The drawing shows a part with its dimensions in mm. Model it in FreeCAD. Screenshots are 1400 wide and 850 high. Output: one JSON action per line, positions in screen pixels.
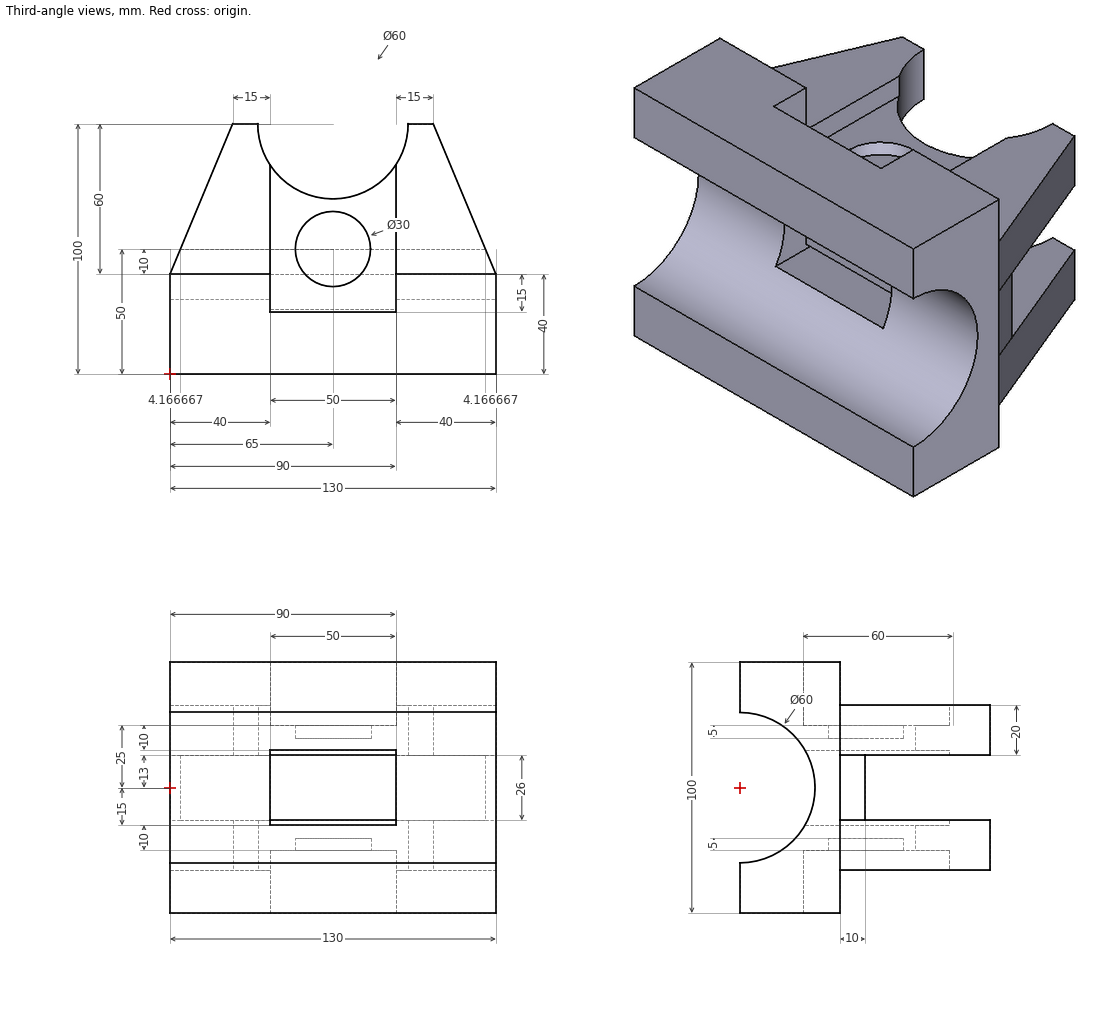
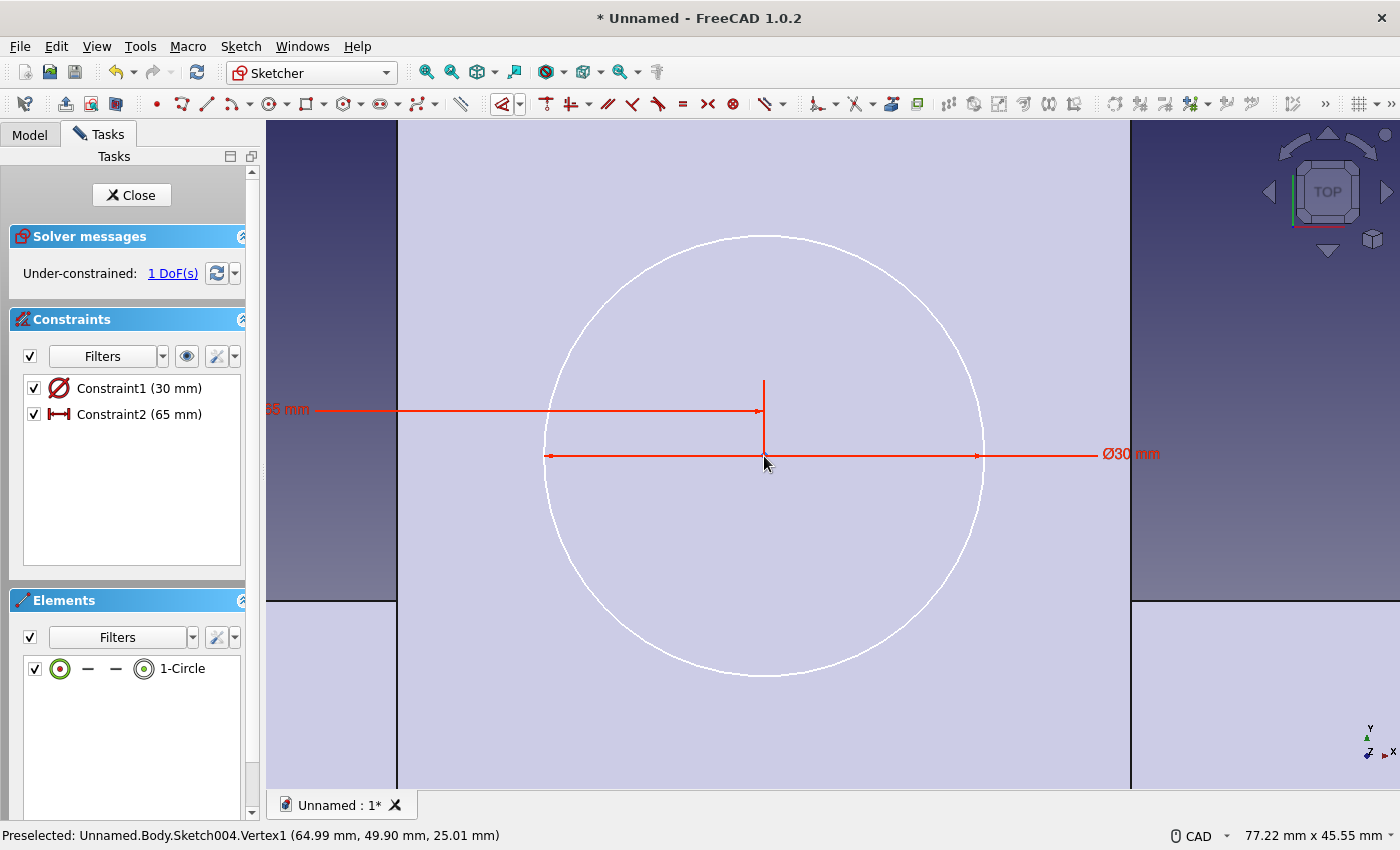
{"action": "left_click", "coordinate": [764, 456]}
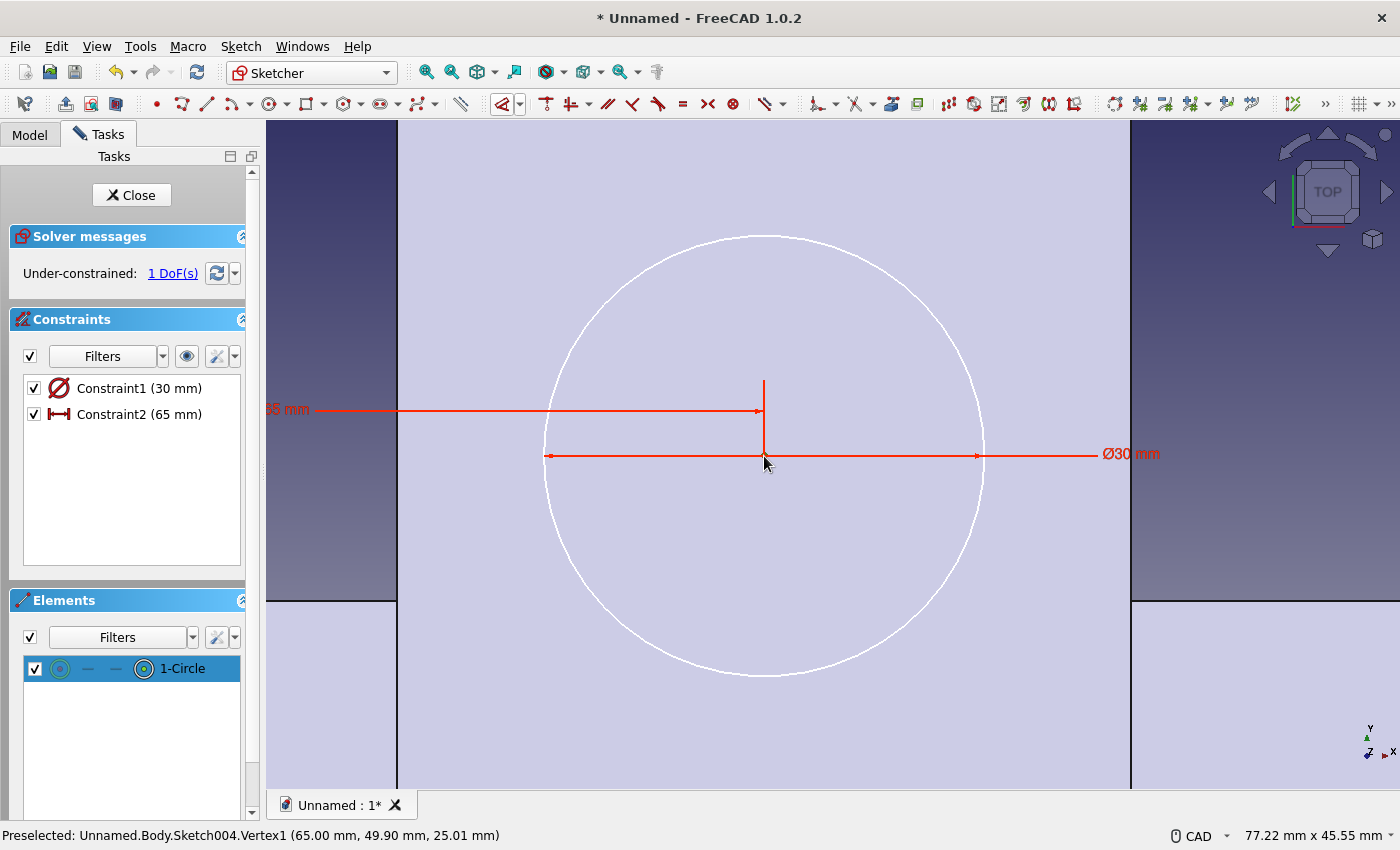
{"action": "key", "text": "i"}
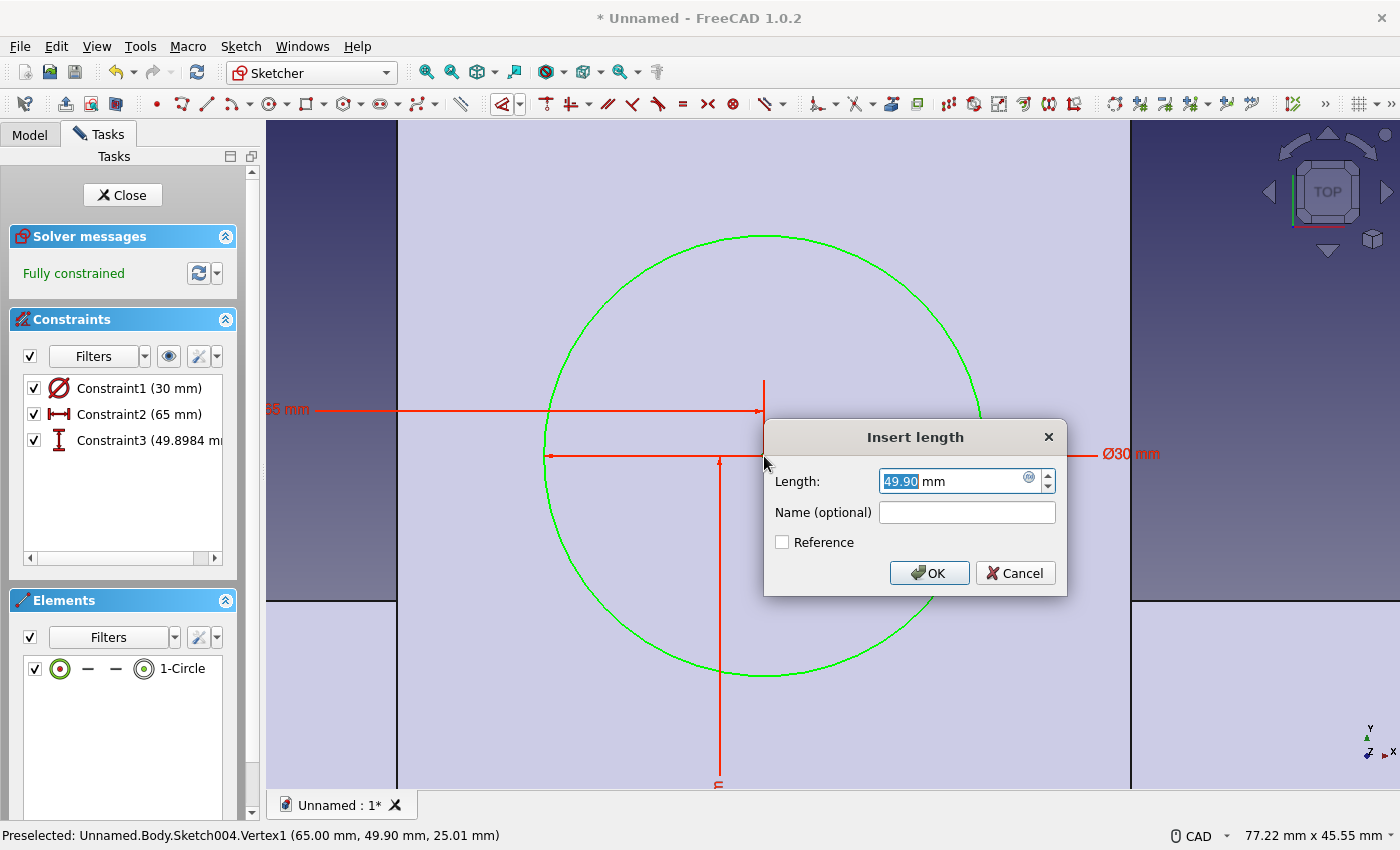
{"action": "type", "text": "50"}
{"action": "key", "text": "Return"}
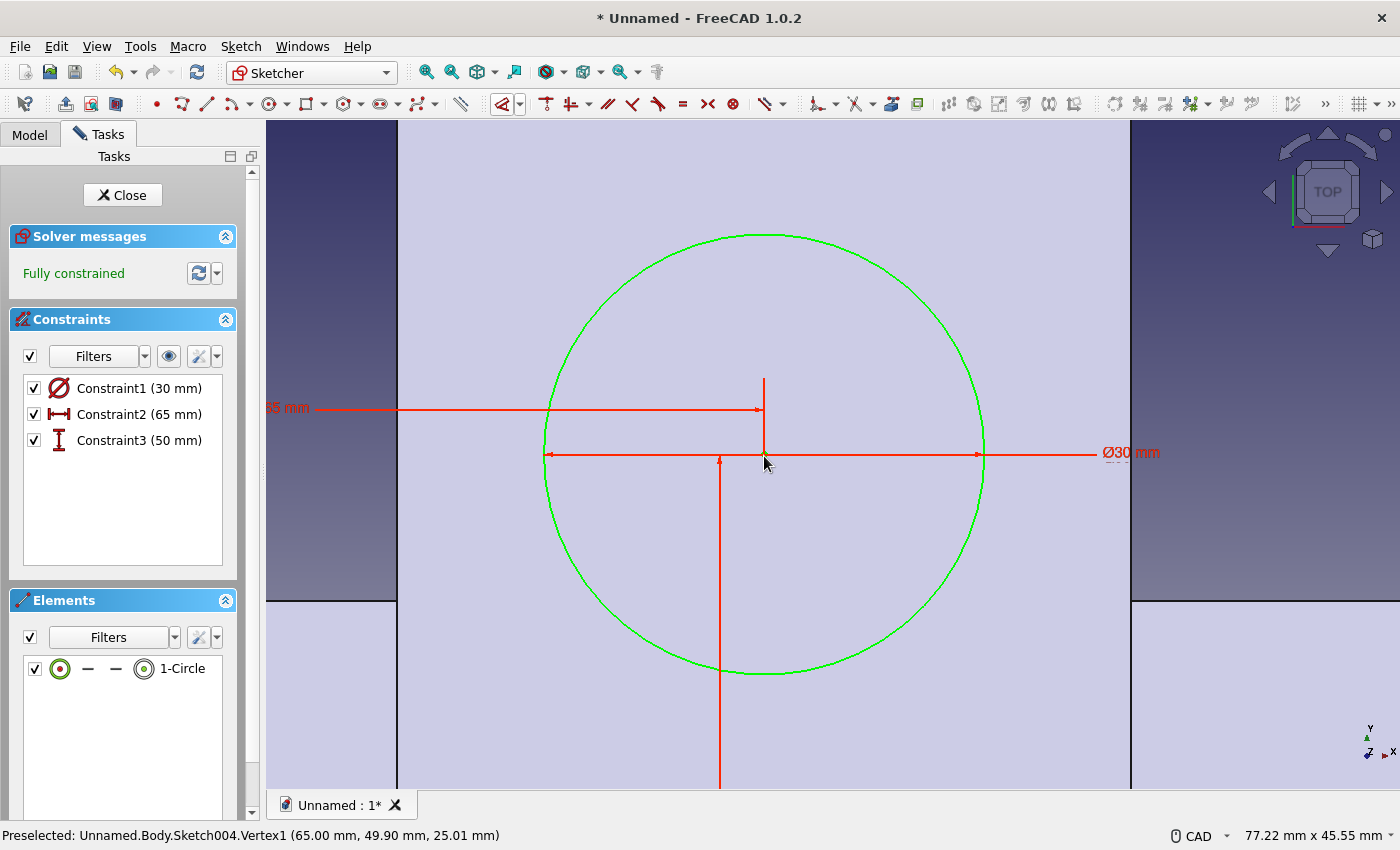
{"action": "left_click", "coordinate": [123, 195]}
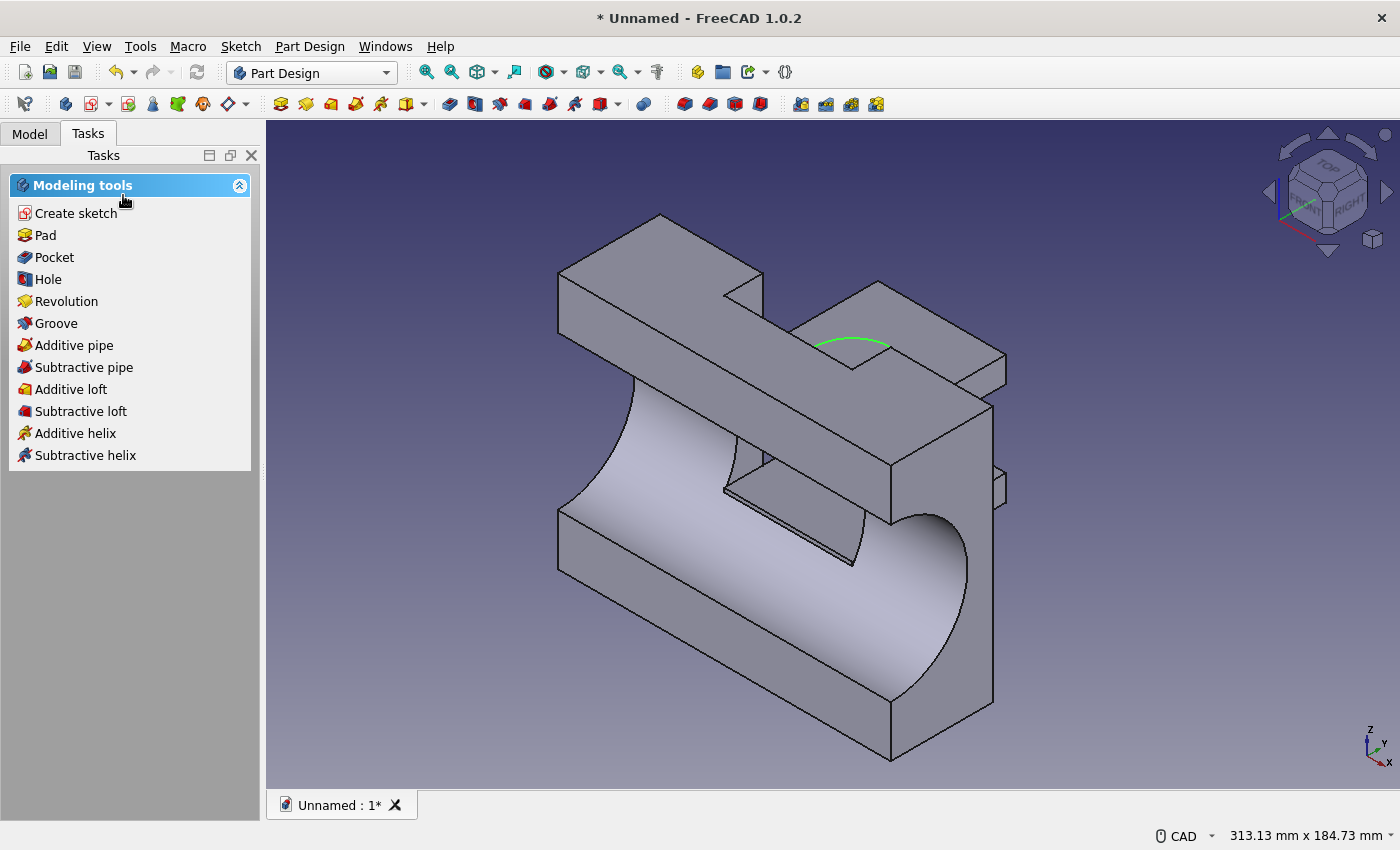
{"action": "left_click", "coordinate": [450, 104]}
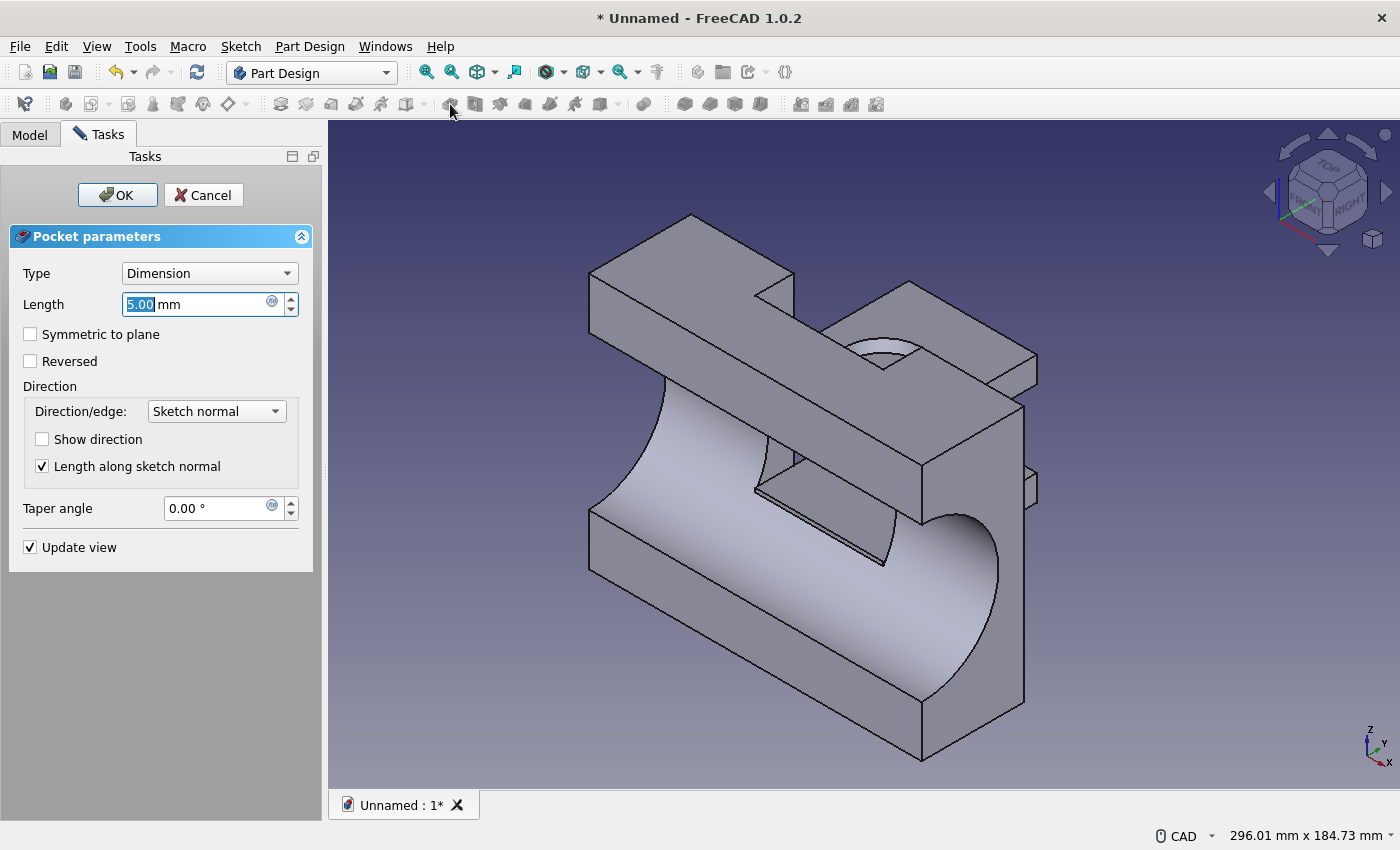
{"action": "type", "text": "5"}
{"action": "key", "text": "Tab"}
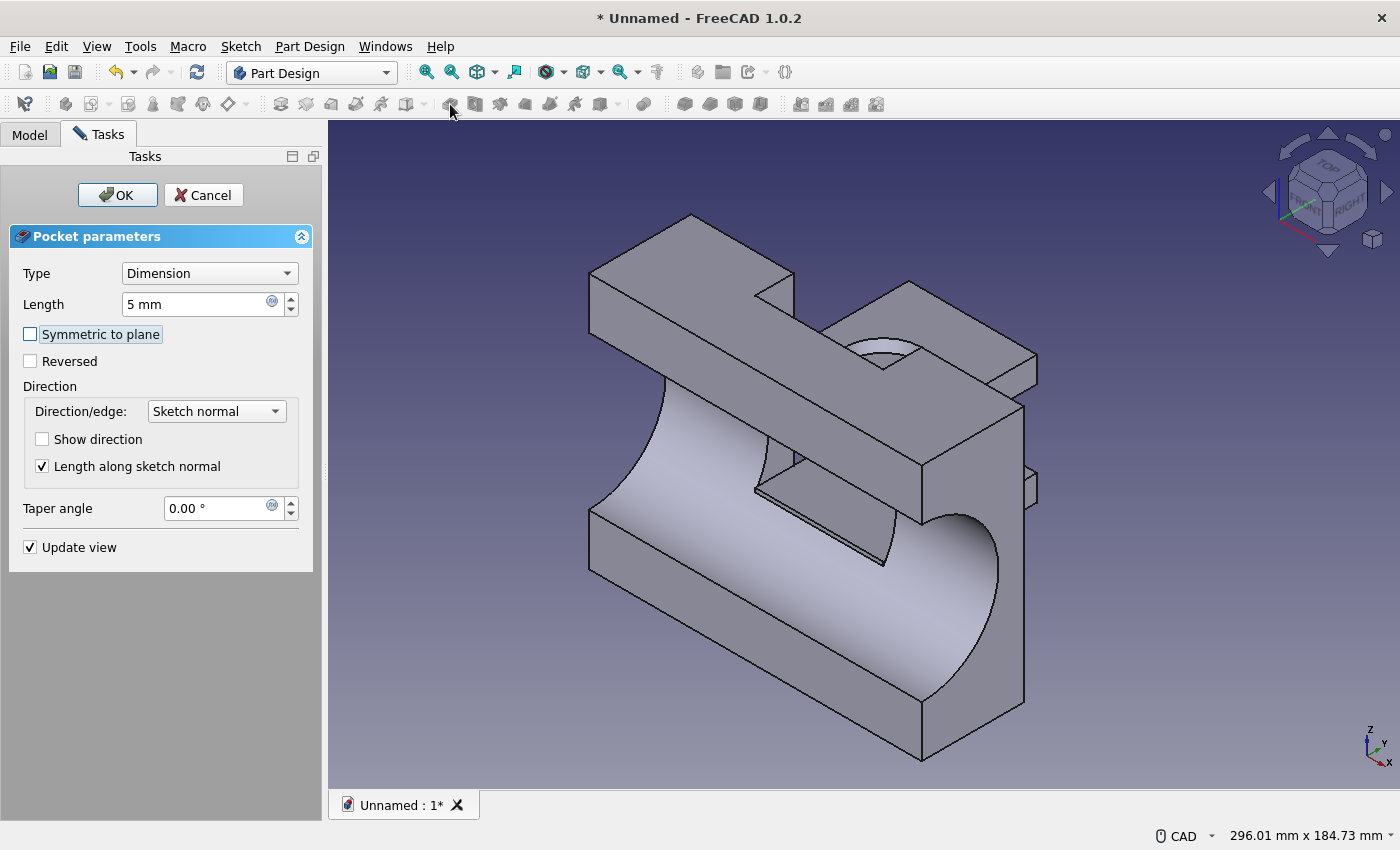
{"action": "left_click", "coordinate": [118, 195]}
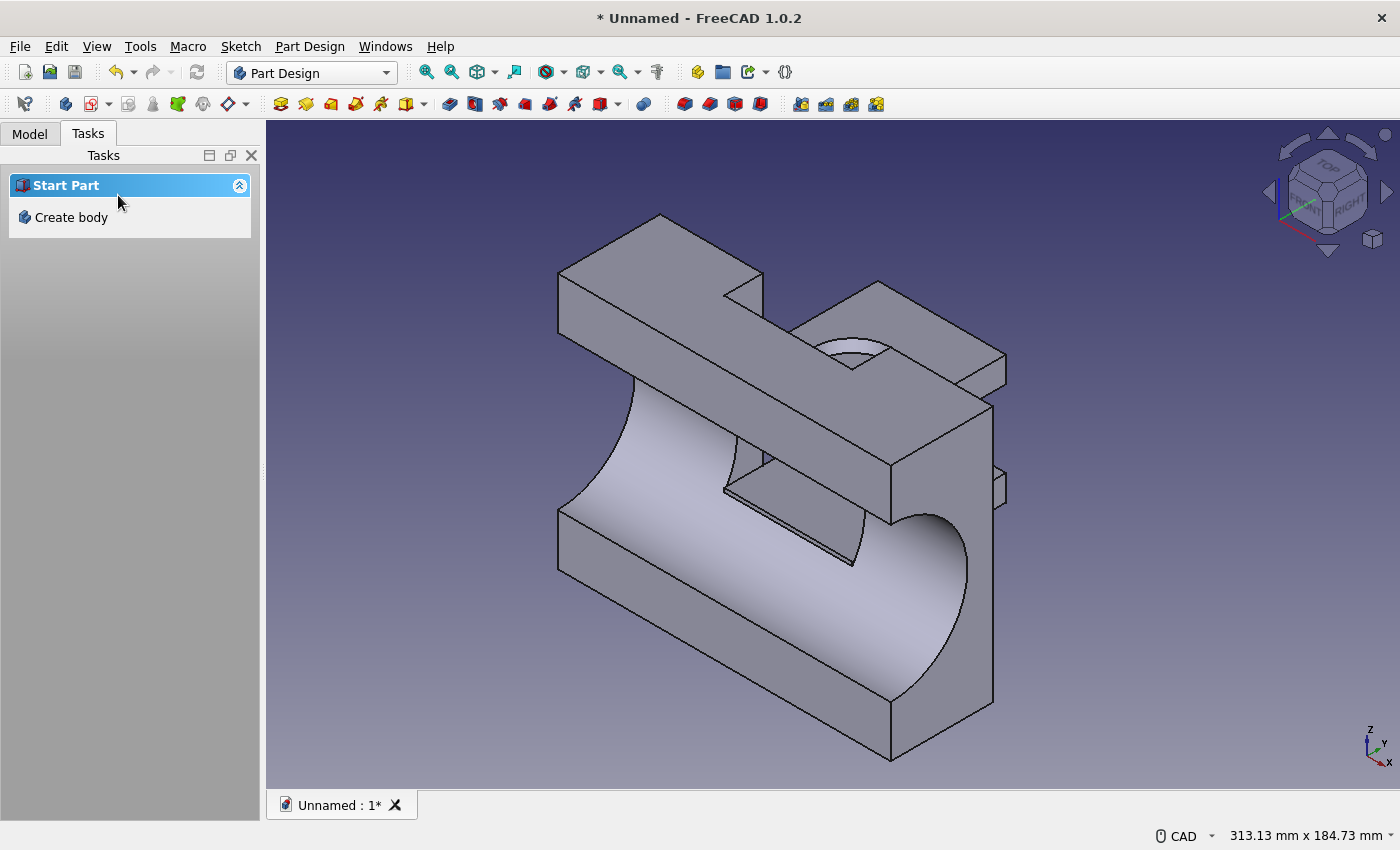
{"action": "left_click", "coordinate": [30, 134]}